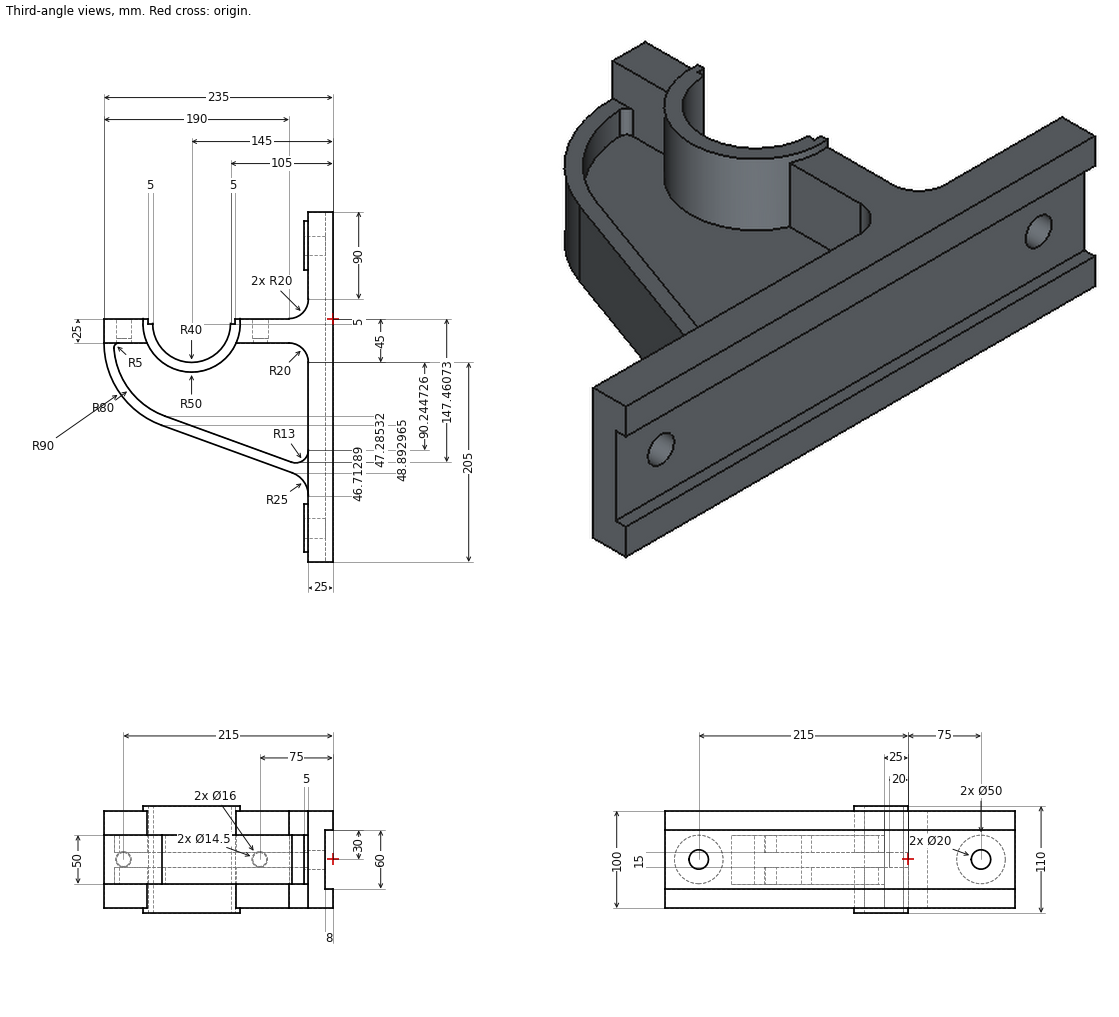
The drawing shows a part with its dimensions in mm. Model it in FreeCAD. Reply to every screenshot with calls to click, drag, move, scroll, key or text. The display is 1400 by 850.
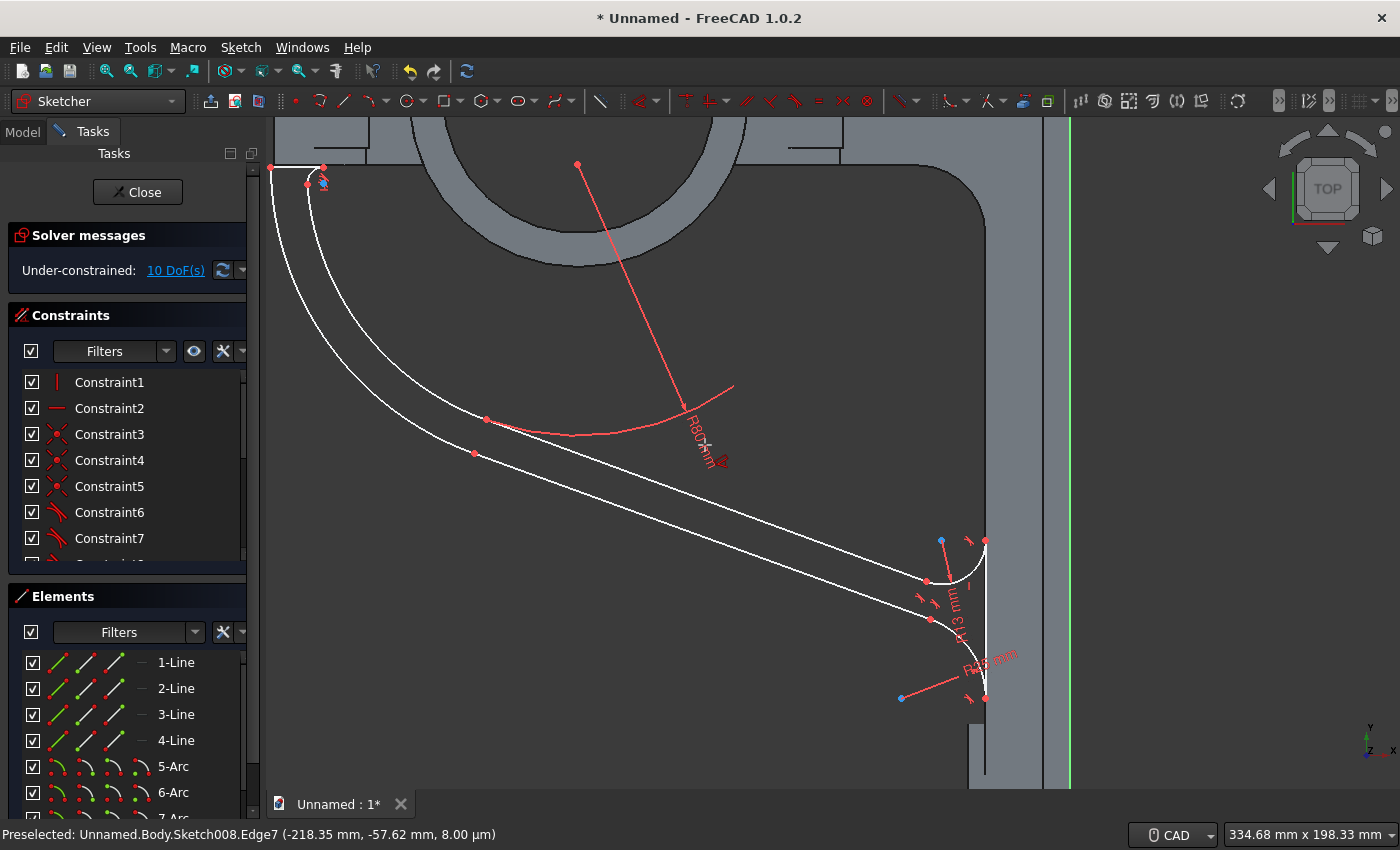
scroll(309, 177, up, 5)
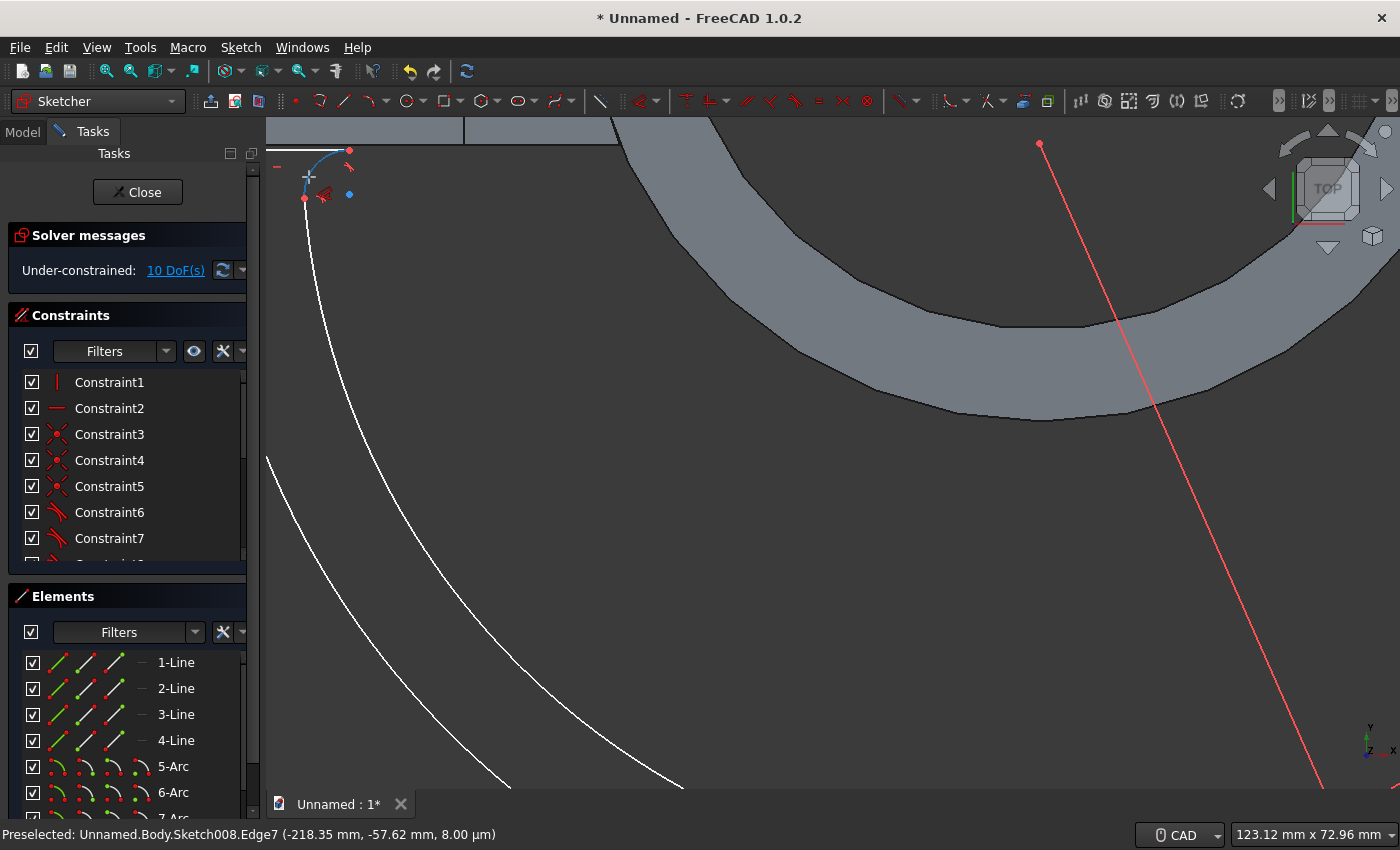
click(308, 177)
click(420, 226)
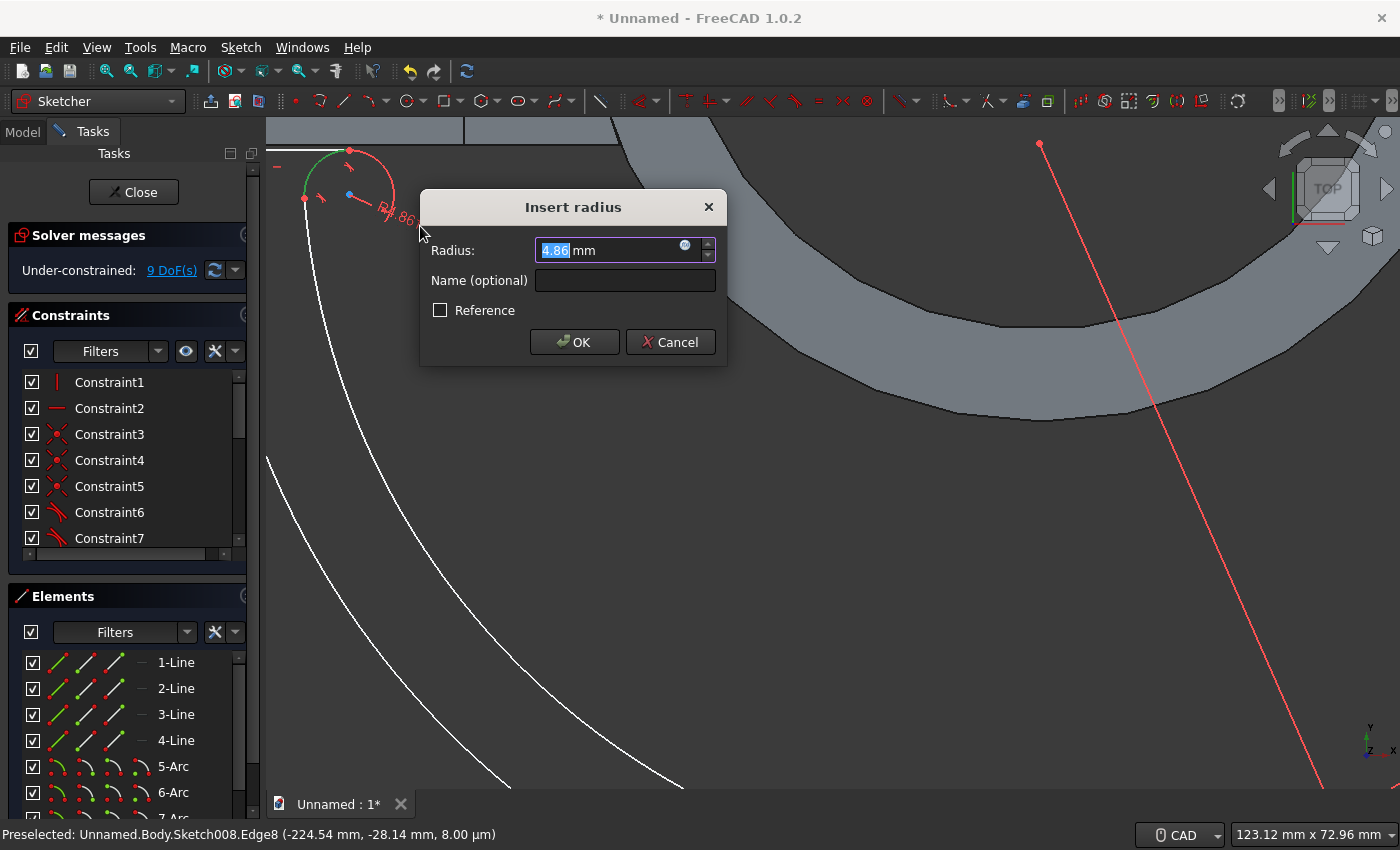
text(5)
key(Return)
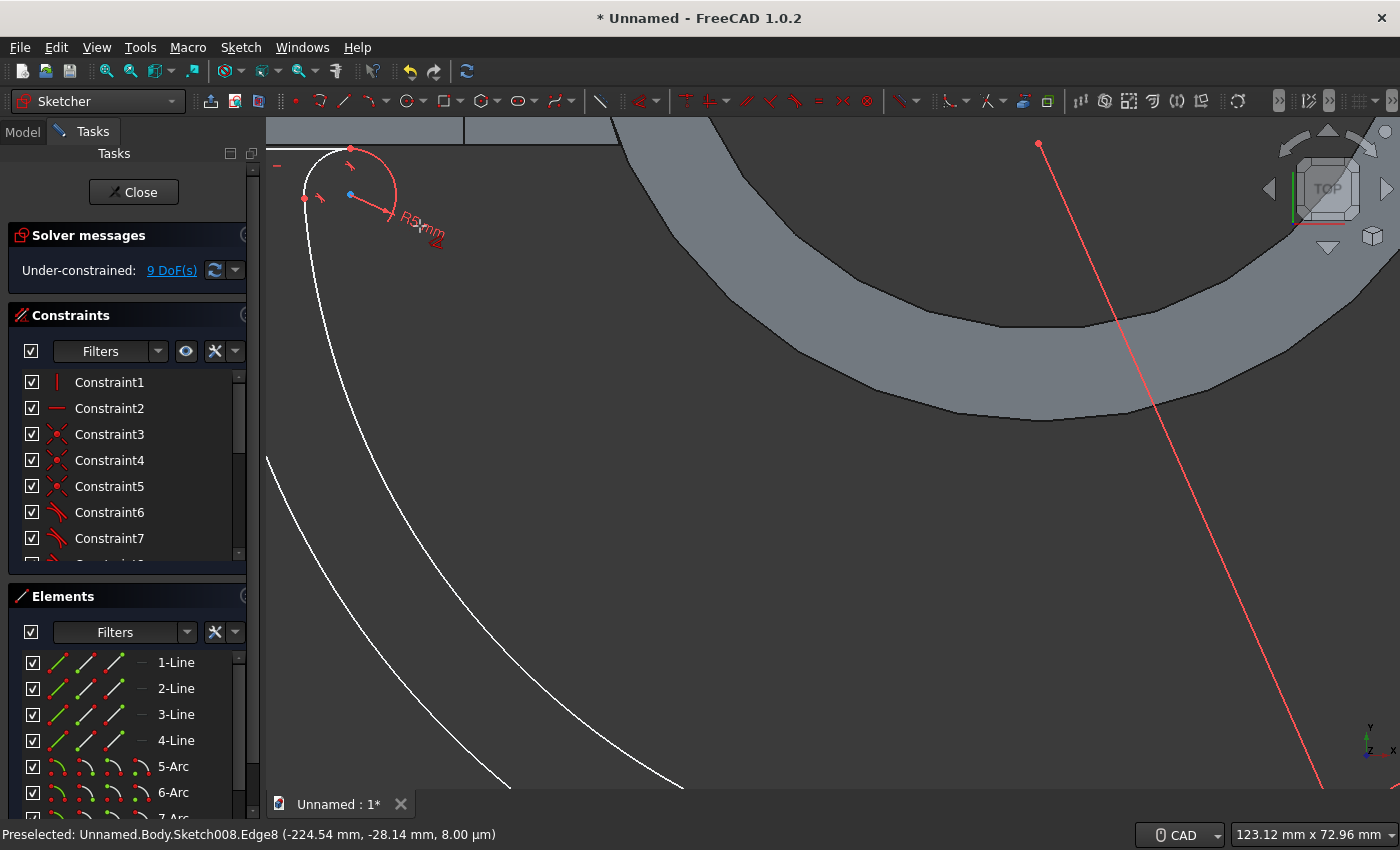
scroll(591, 355, down, 7)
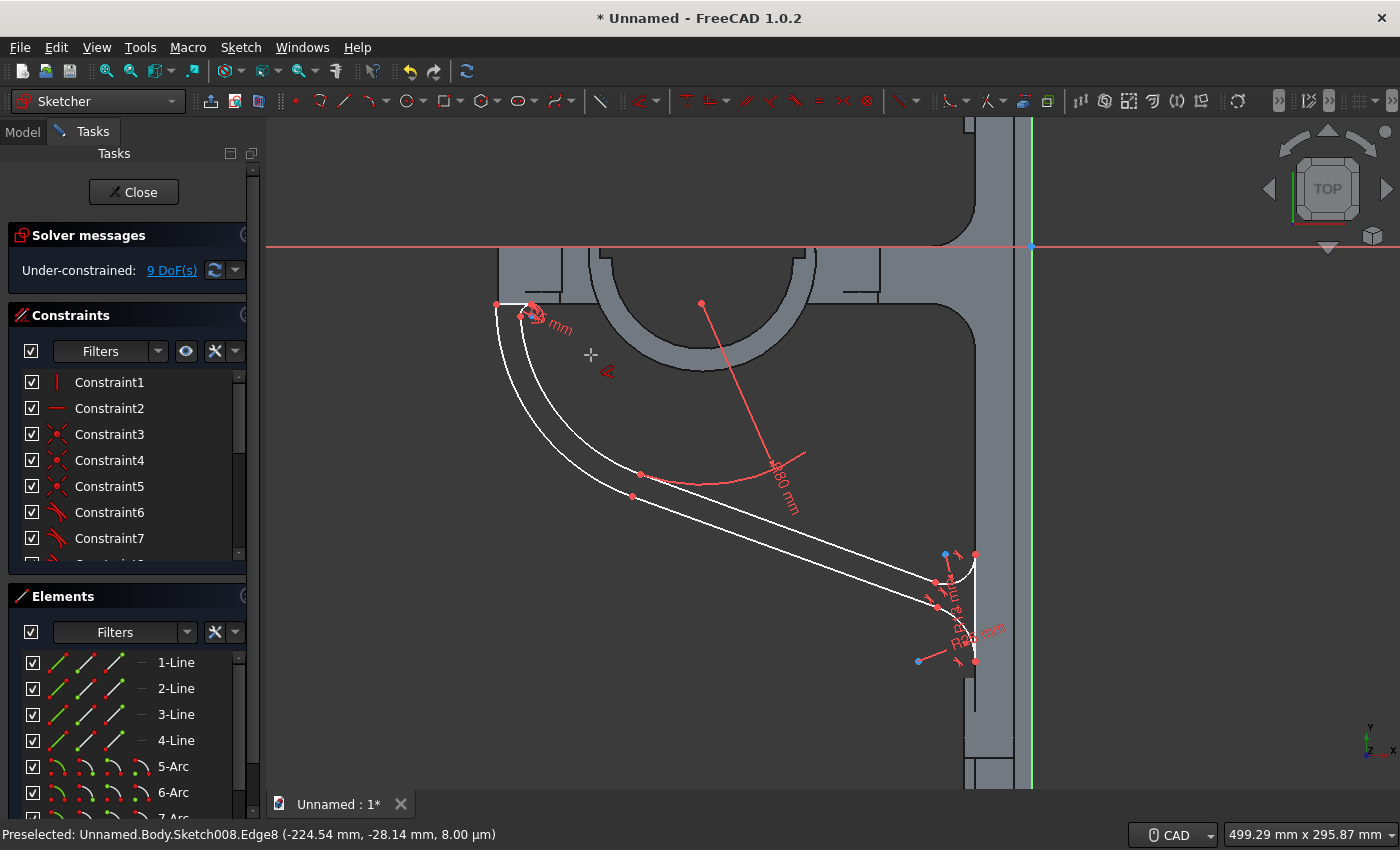
click(534, 422)
click(508, 441)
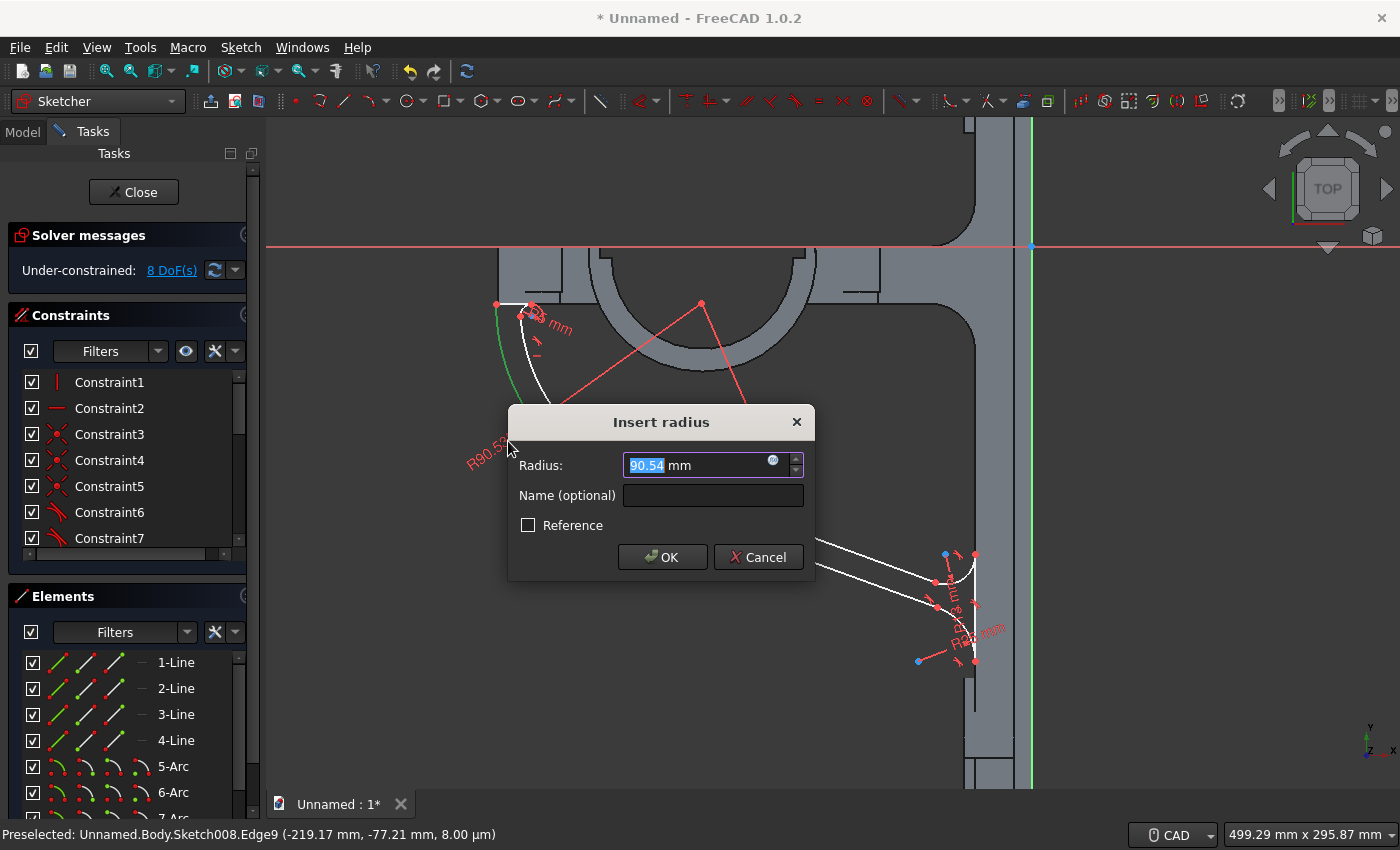
text(90)
key(Return)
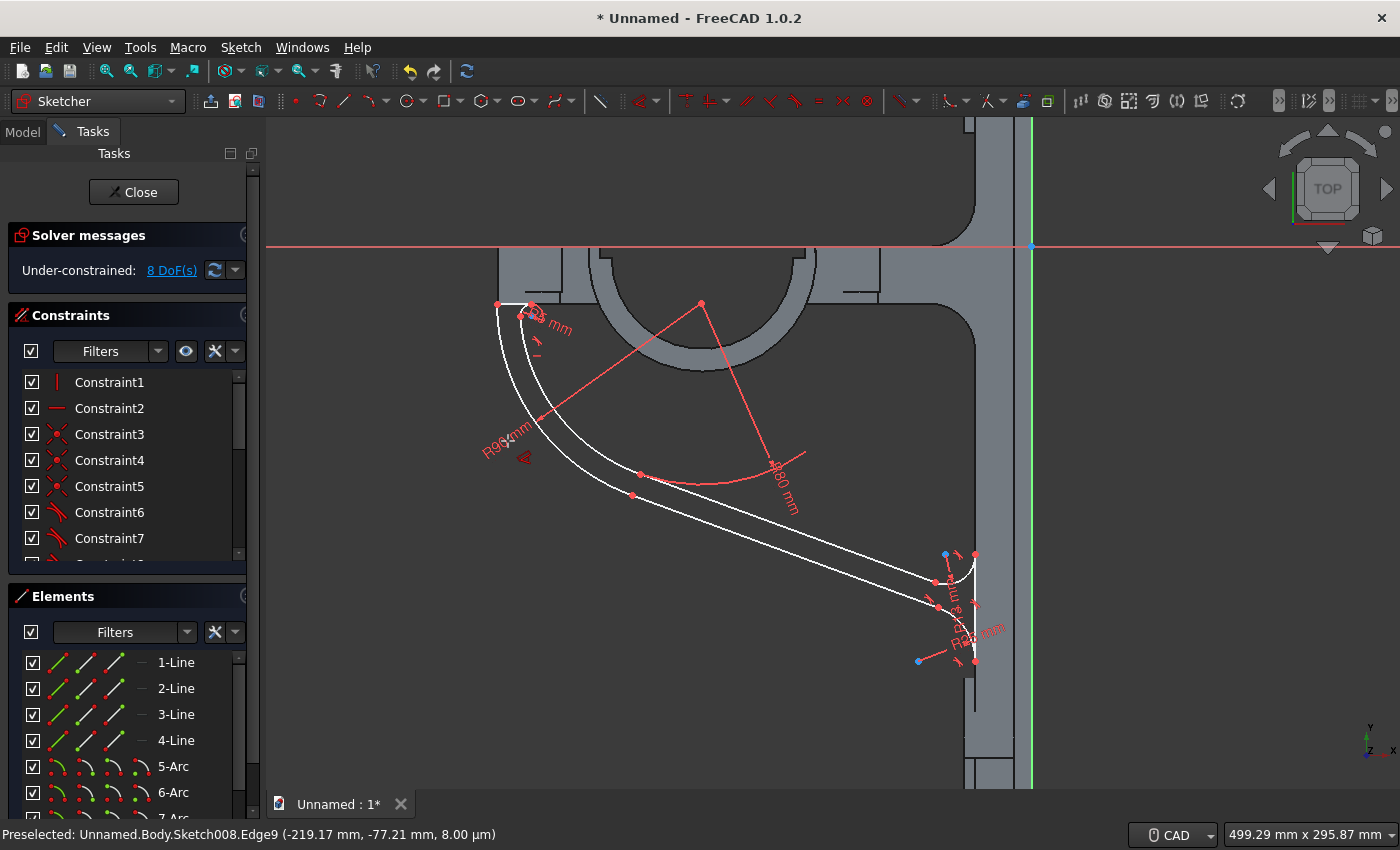
click(975, 661)
click(1004, 695)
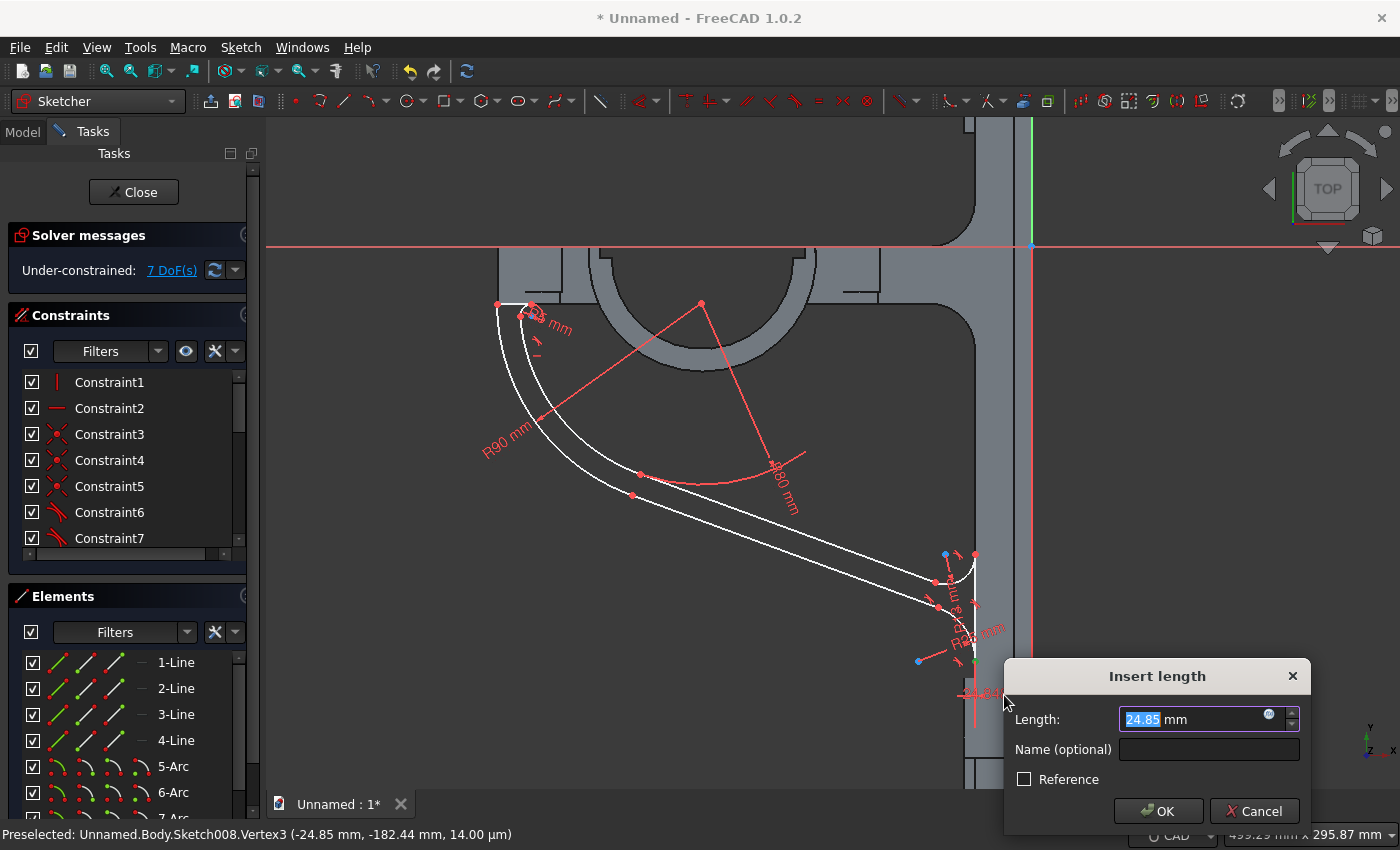
text(25)
key(Return)